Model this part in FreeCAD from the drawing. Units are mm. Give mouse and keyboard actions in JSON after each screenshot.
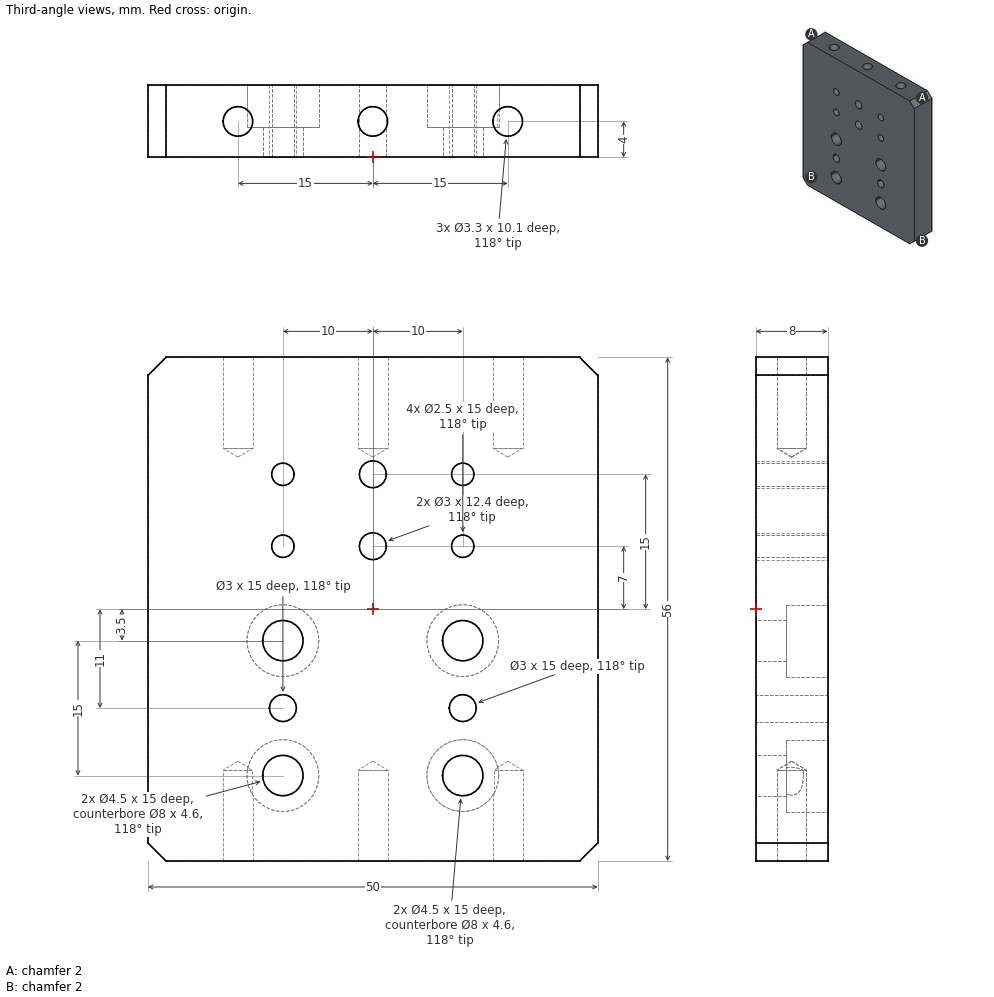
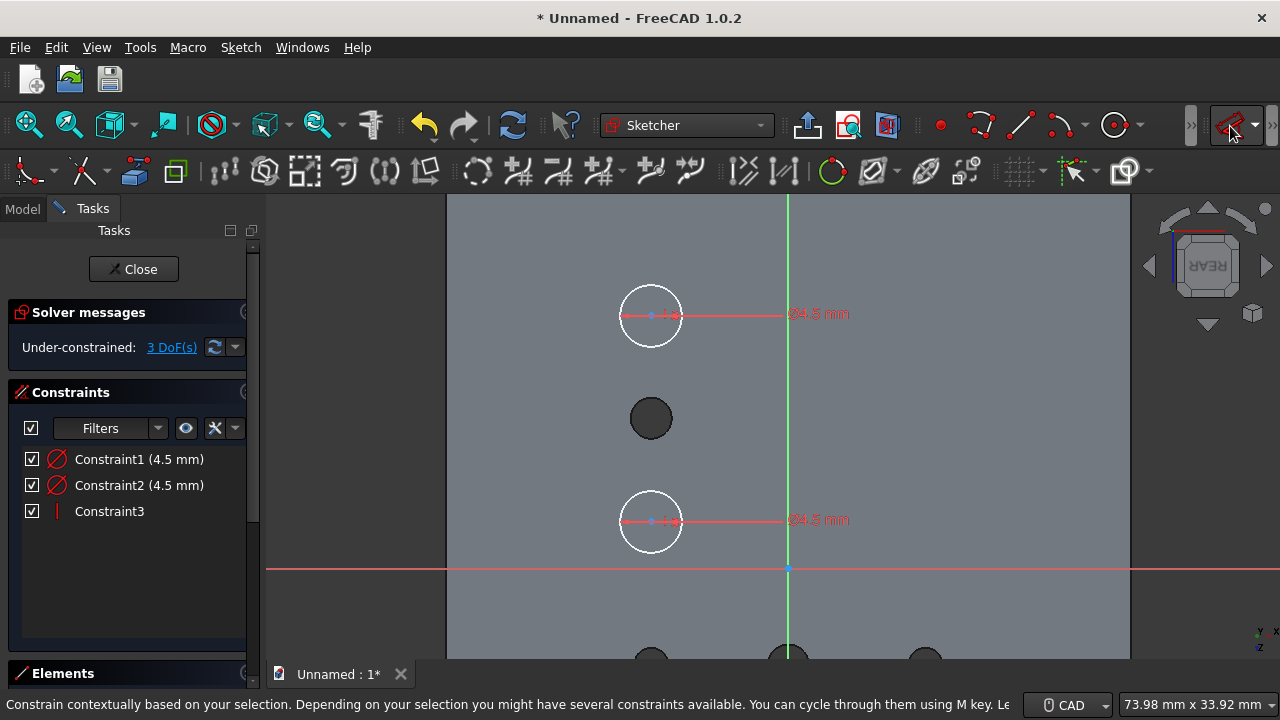
{"action": "left_click", "coordinate": [651, 316]}
{"action": "left_click", "coordinate": [720, 603]}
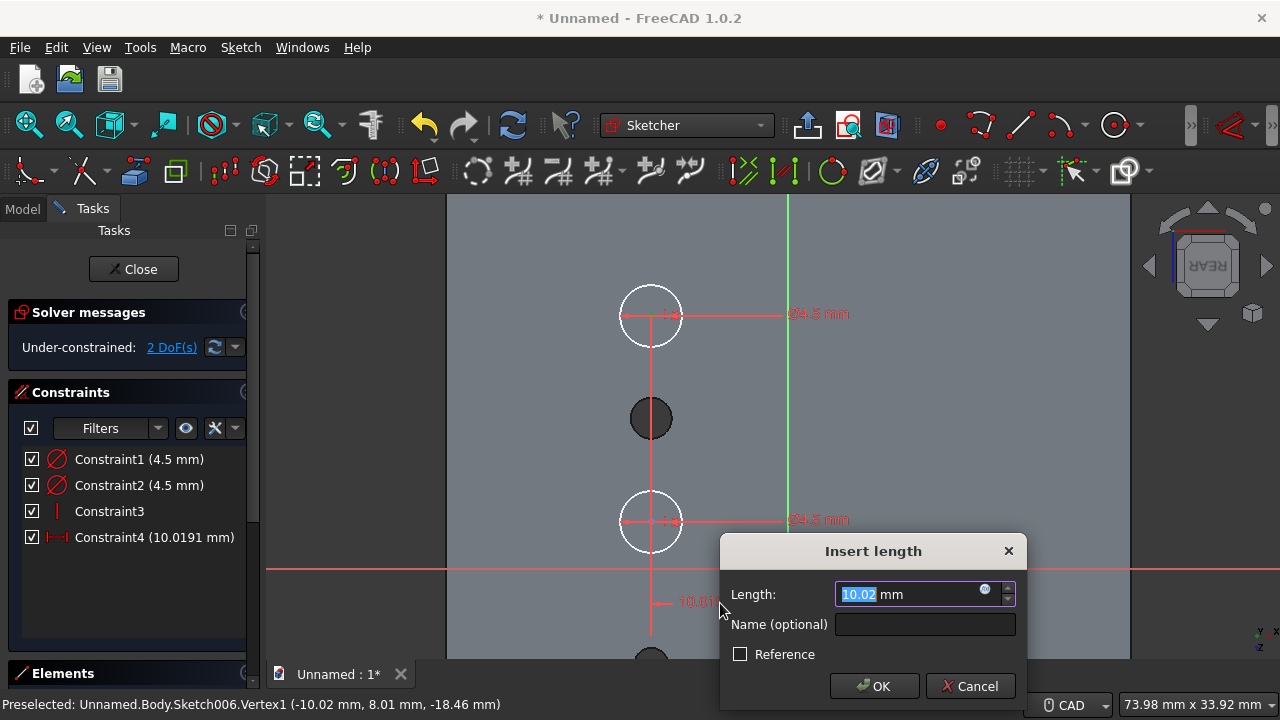
{"action": "type", "text": "10"}
{"action": "key", "text": "Return"}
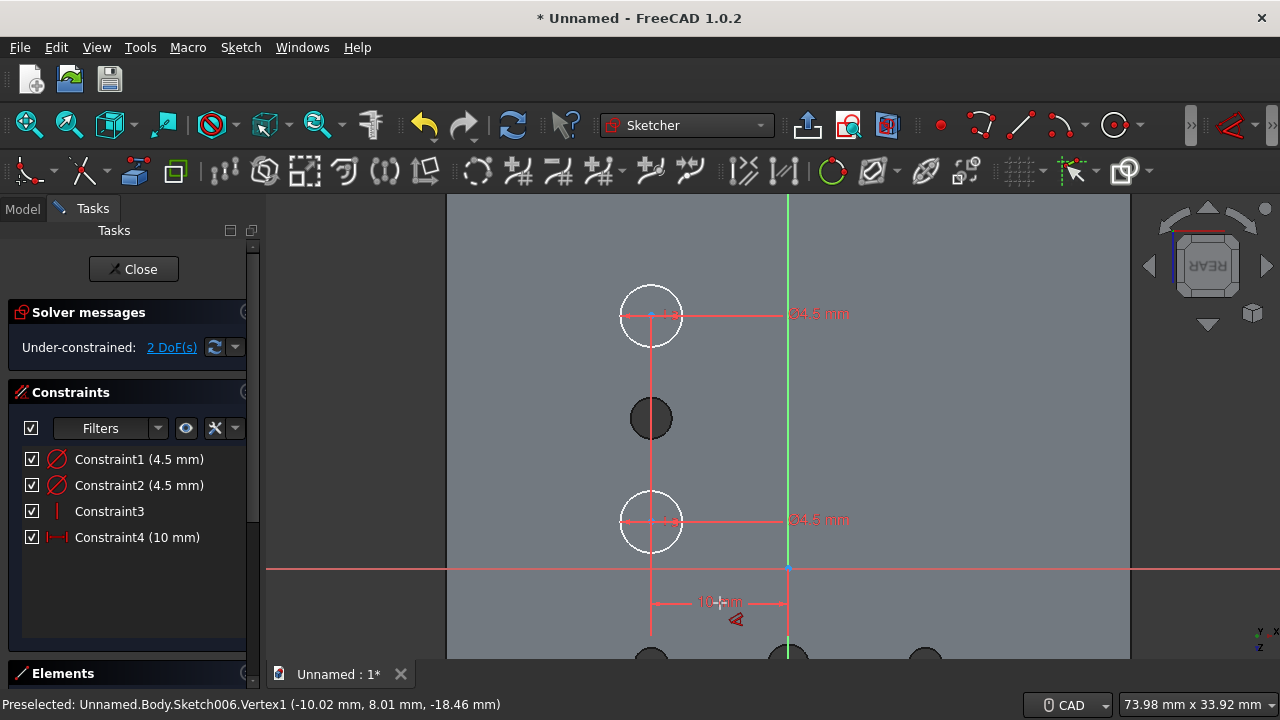
{"action": "left_click", "coordinate": [651, 522]}
{"action": "left_click", "coordinate": [822, 545]}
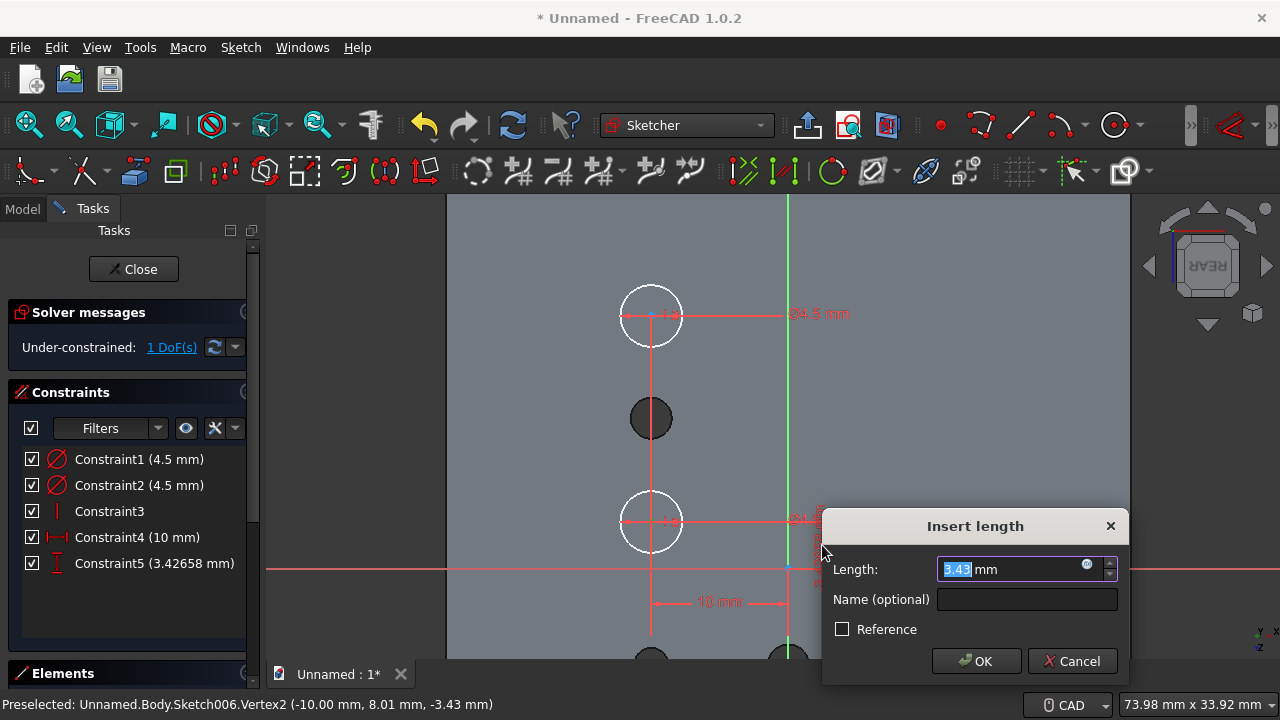
{"action": "type", "text": "3.5"}
{"action": "key", "text": "Return"}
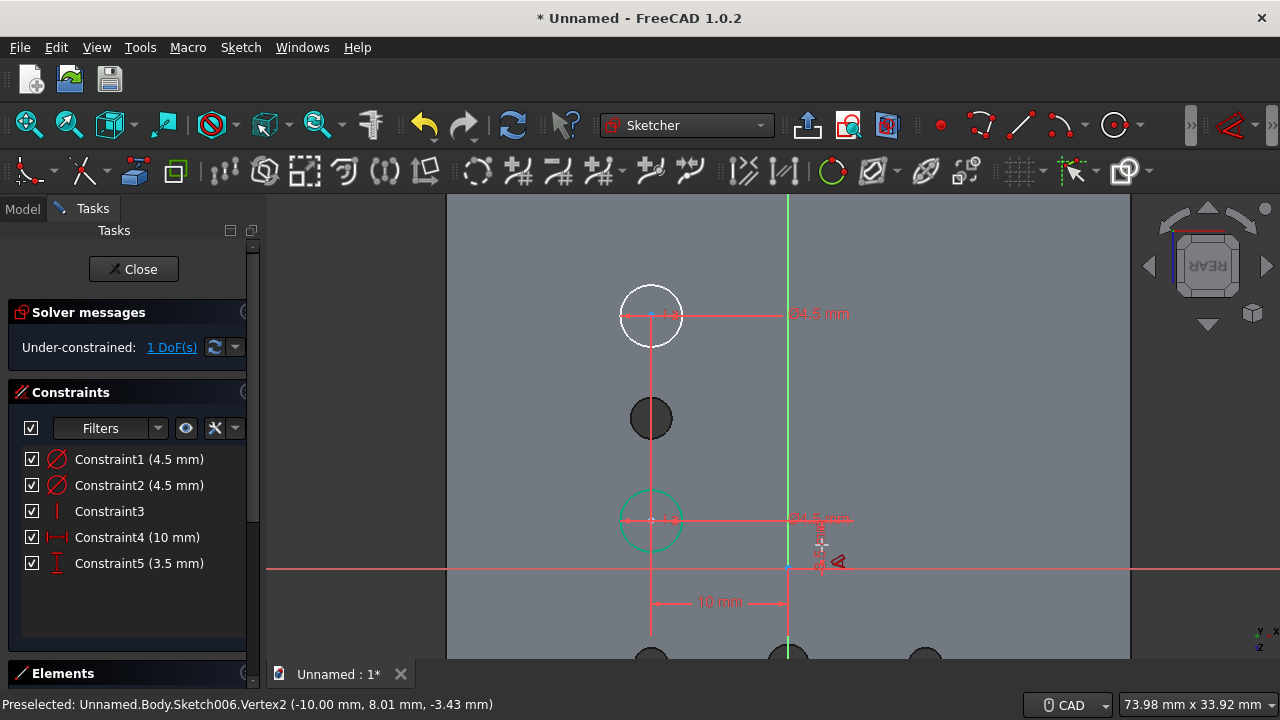
{"action": "left_click", "coordinate": [651, 316]}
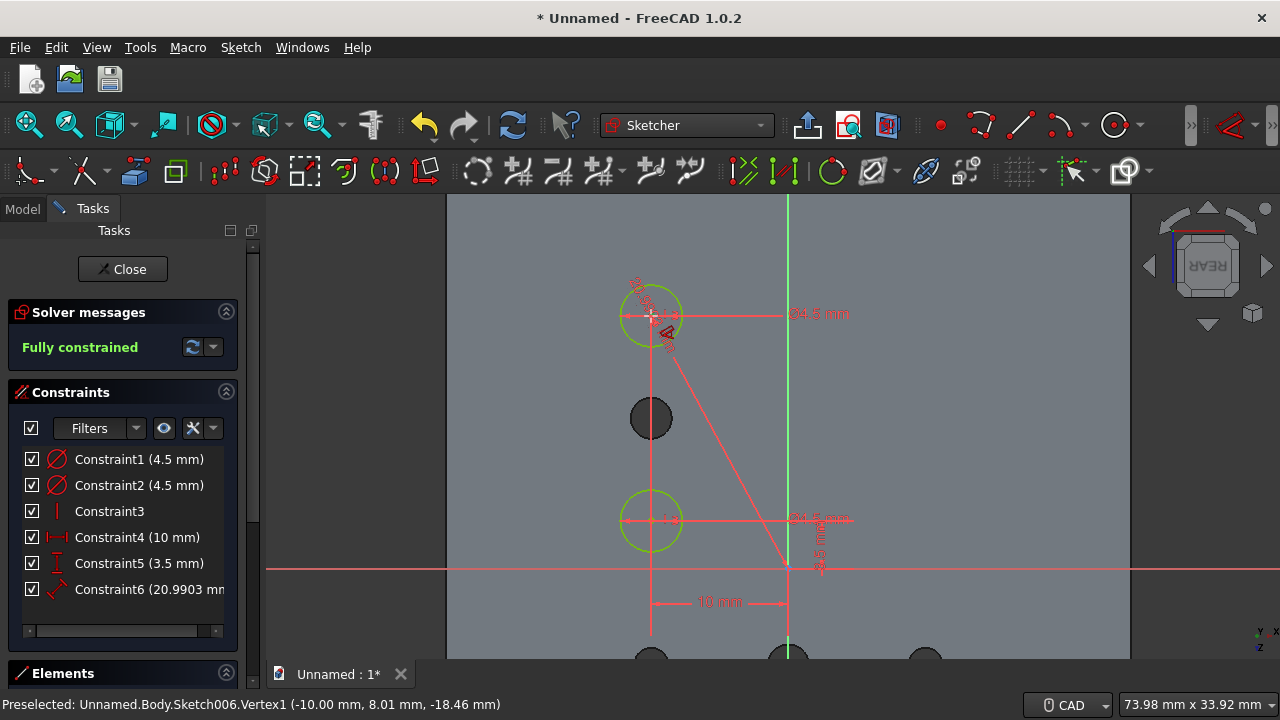
{"action": "left_click", "coordinate": [651, 521]}
{"action": "left_click", "coordinate": [617, 418]}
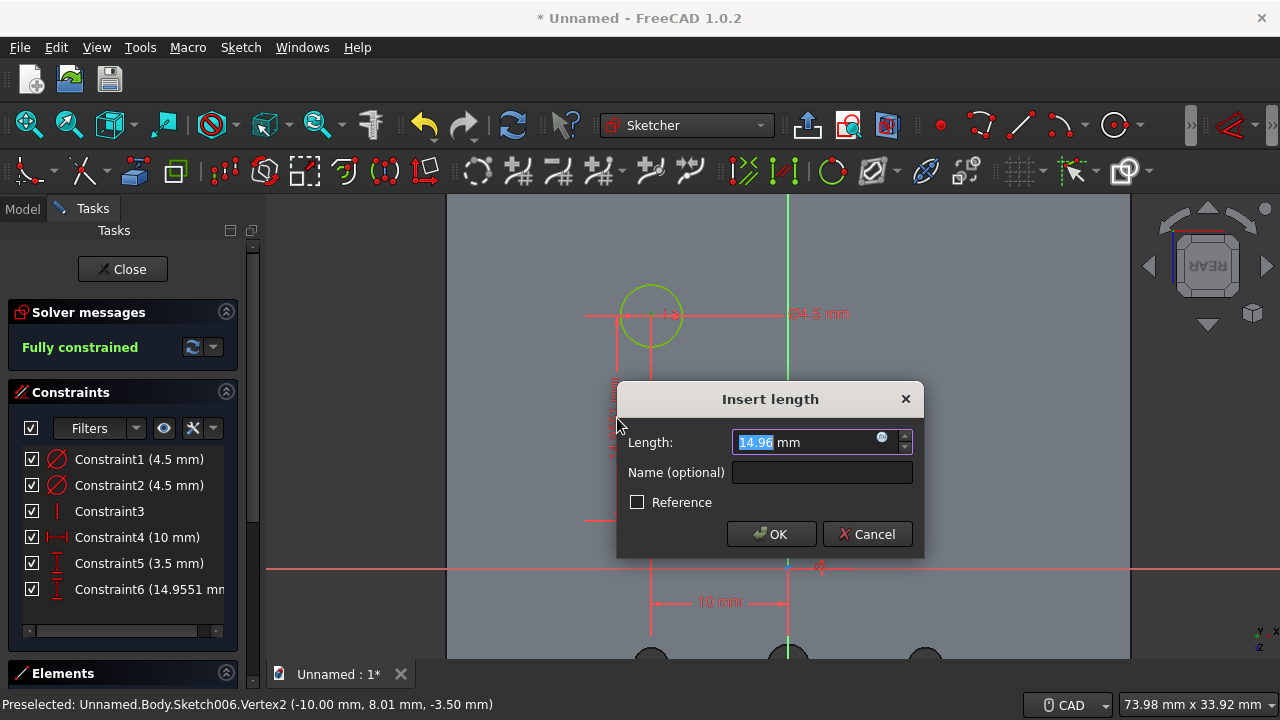
{"action": "type", "text": "15"}
{"action": "key", "text": "Return"}
{"action": "key", "text": "Escape"}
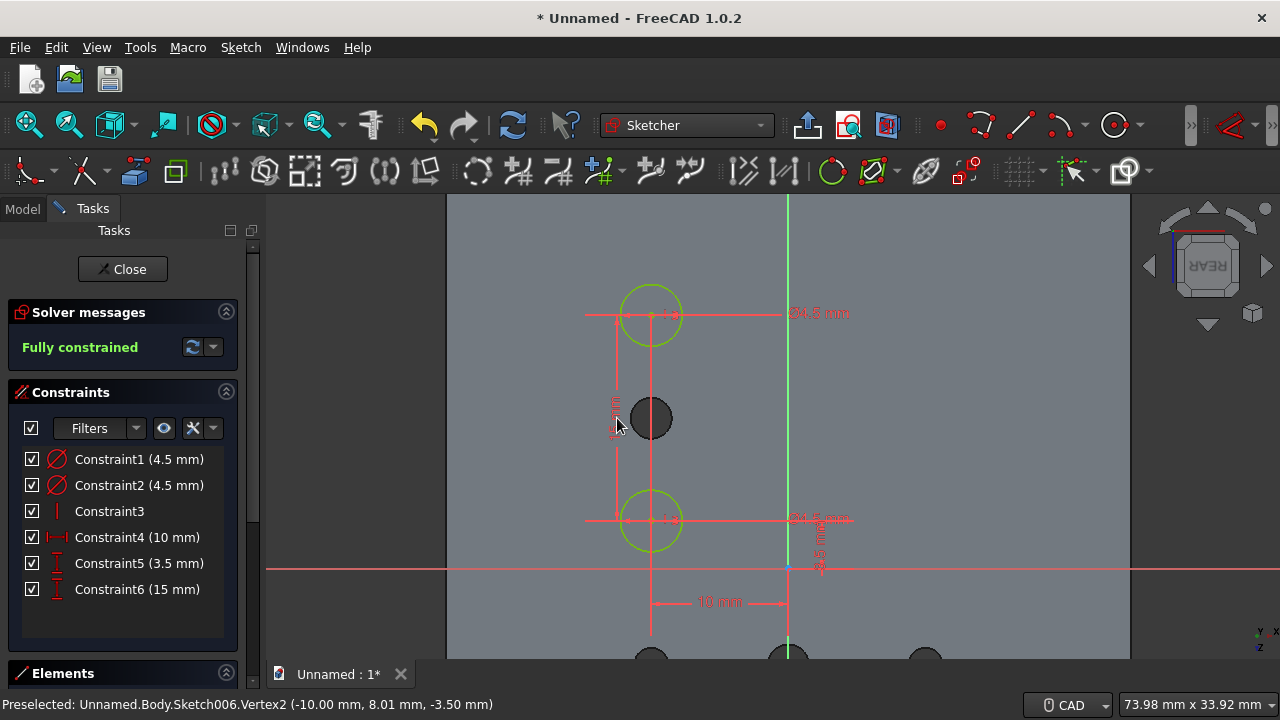
{"action": "left_click", "coordinate": [123, 269]}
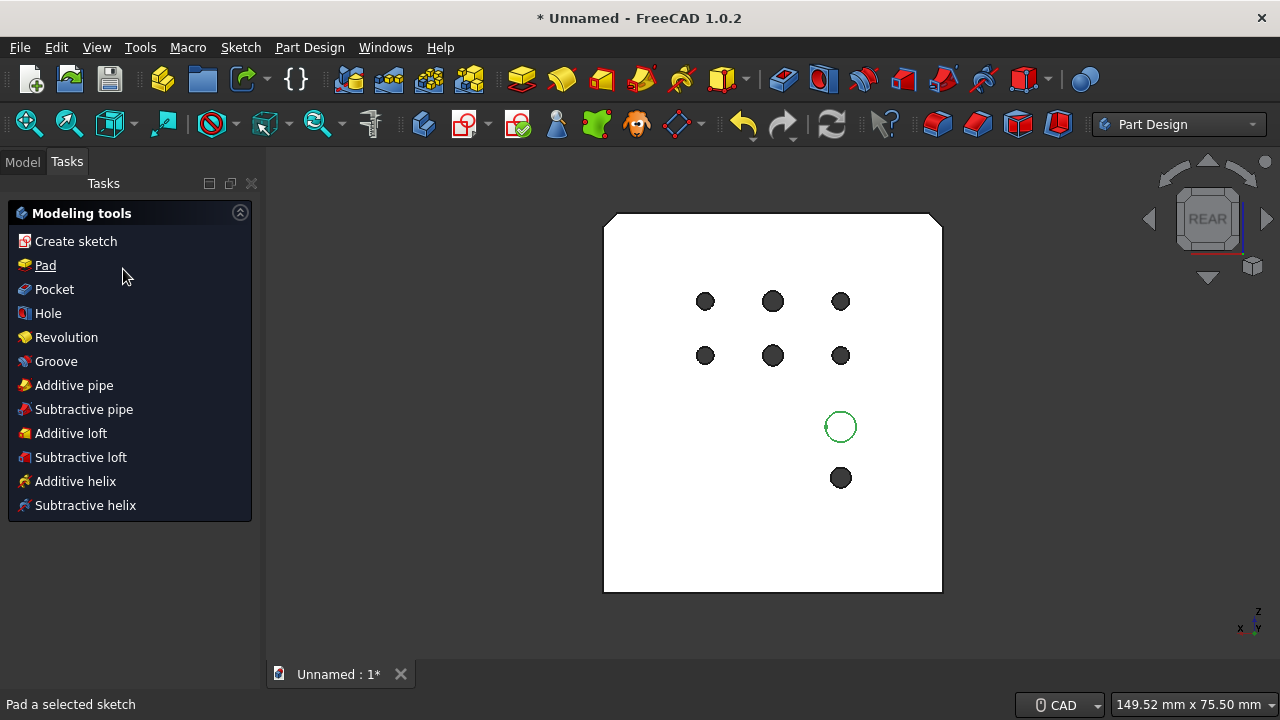
{"action": "left_click", "coordinate": [824, 80]}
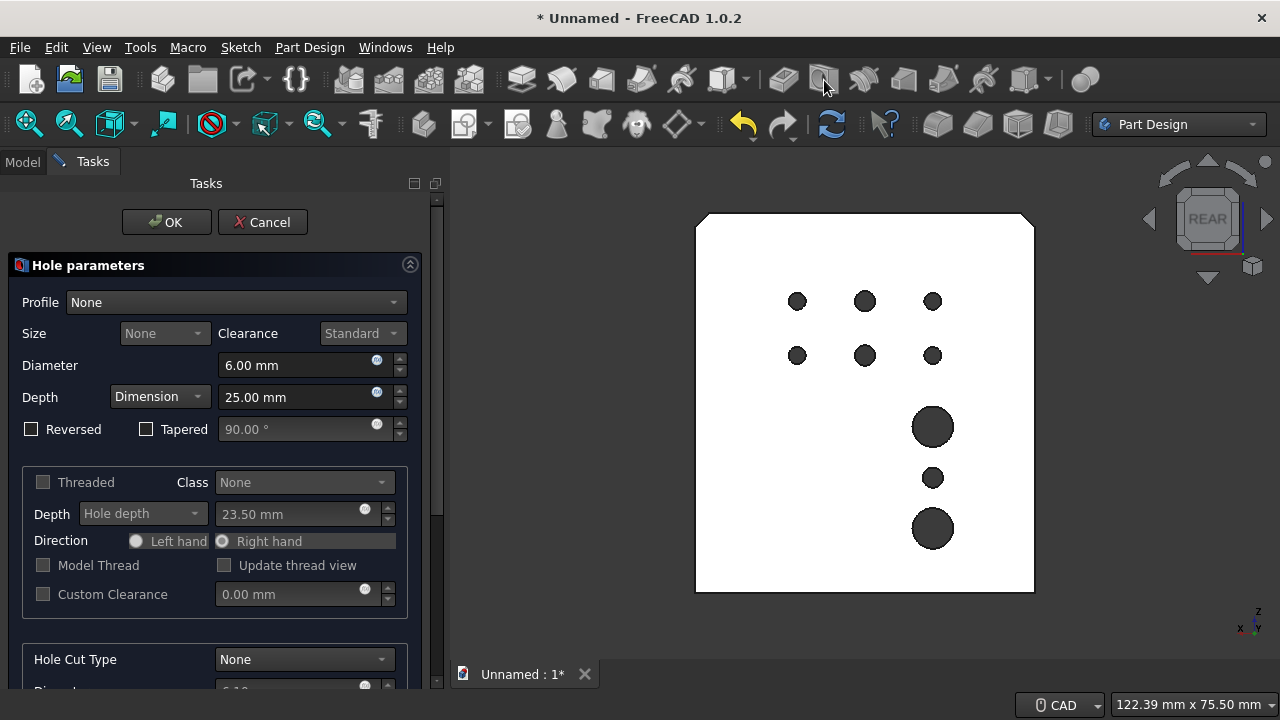
{"action": "triple_click", "coordinate": [305, 365]}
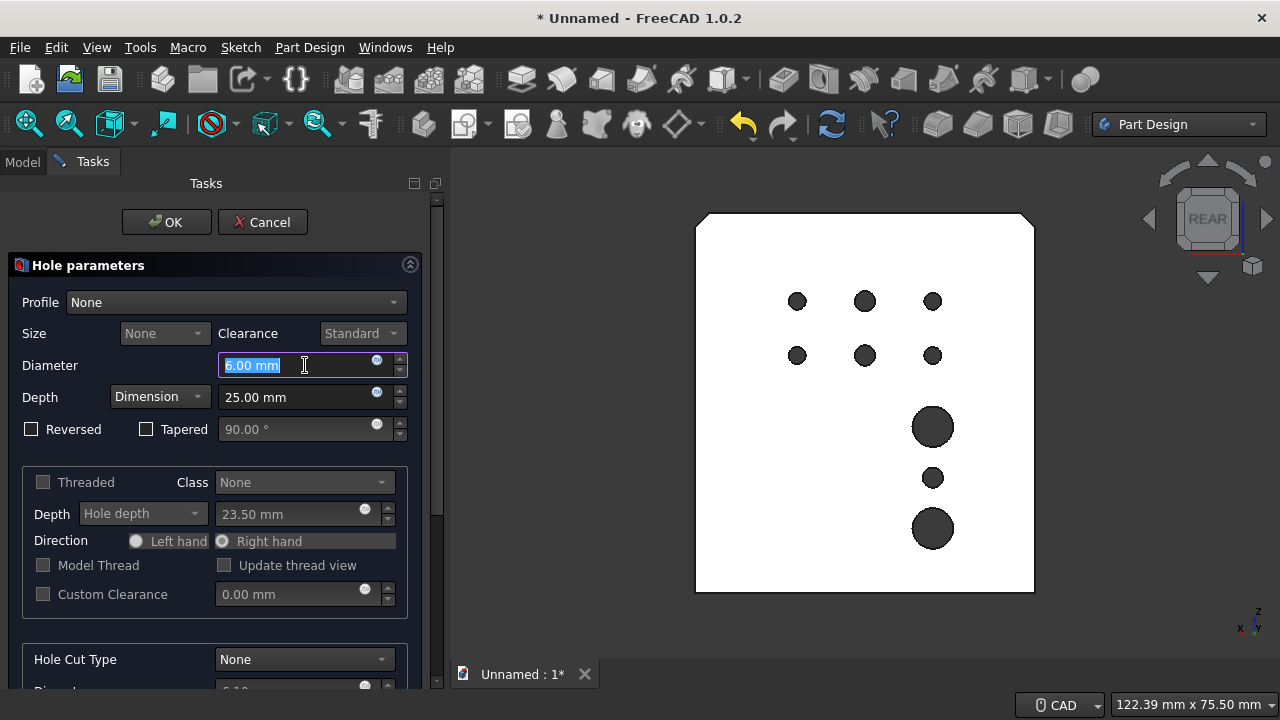
{"action": "type", "text": "4.5"}
{"action": "key", "text": "Tab"}